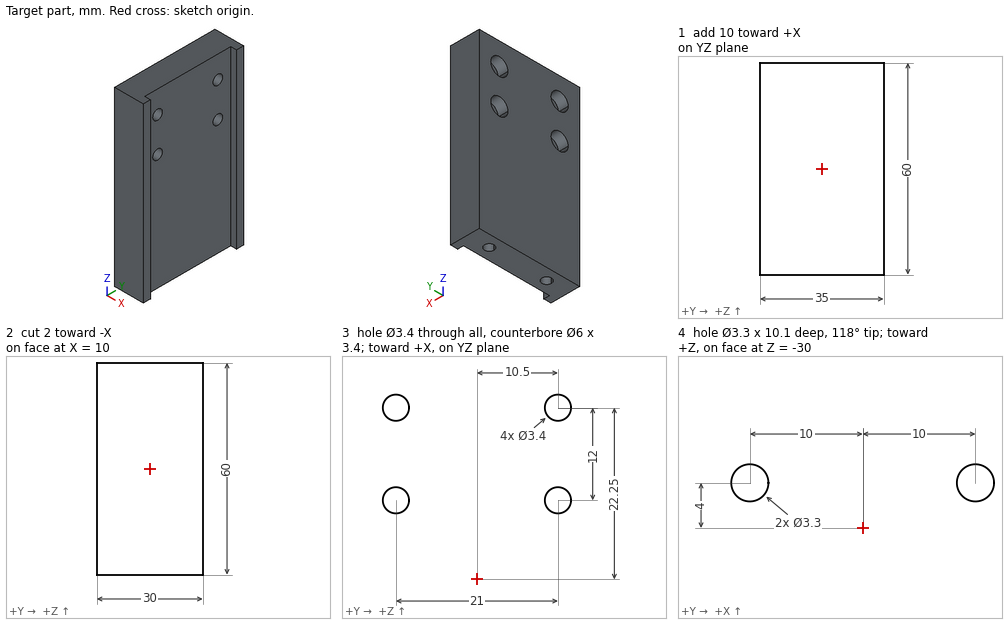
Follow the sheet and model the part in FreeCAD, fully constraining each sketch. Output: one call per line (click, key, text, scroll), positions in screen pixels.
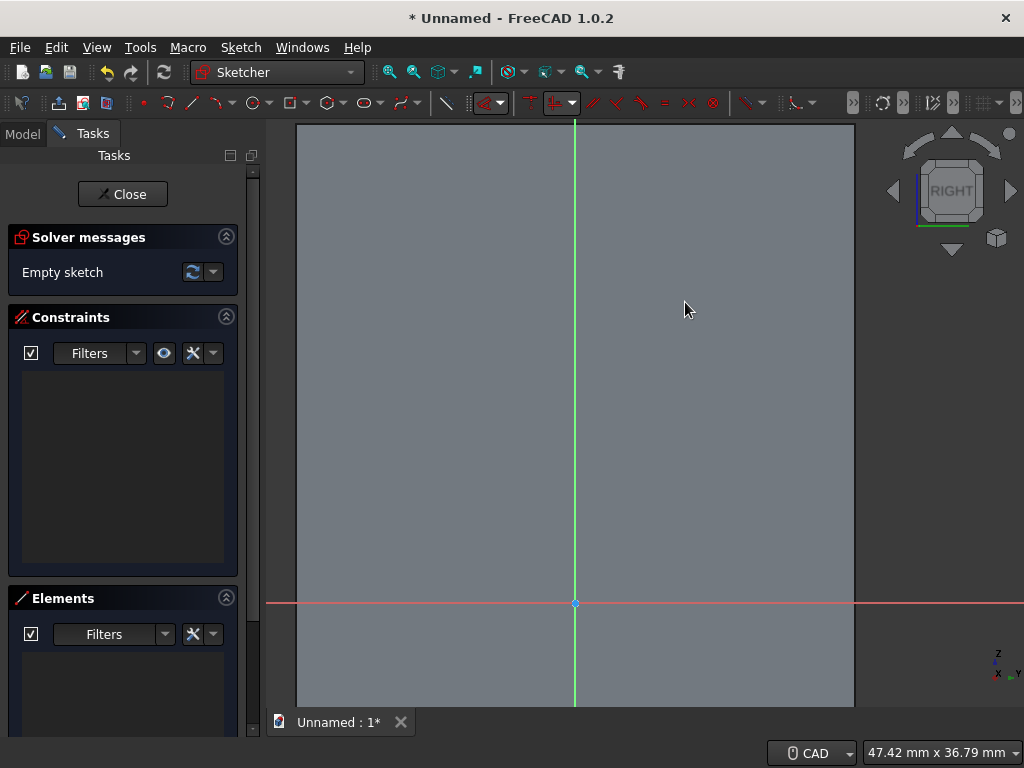
click(254, 104)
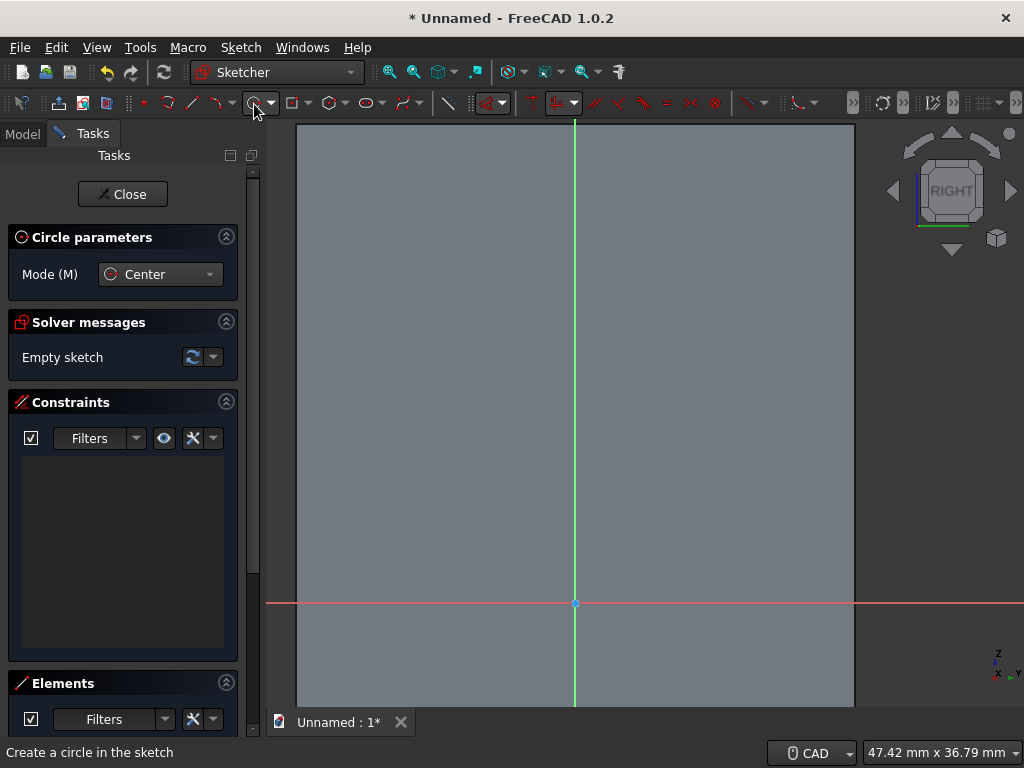
click(743, 248)
move(762, 228)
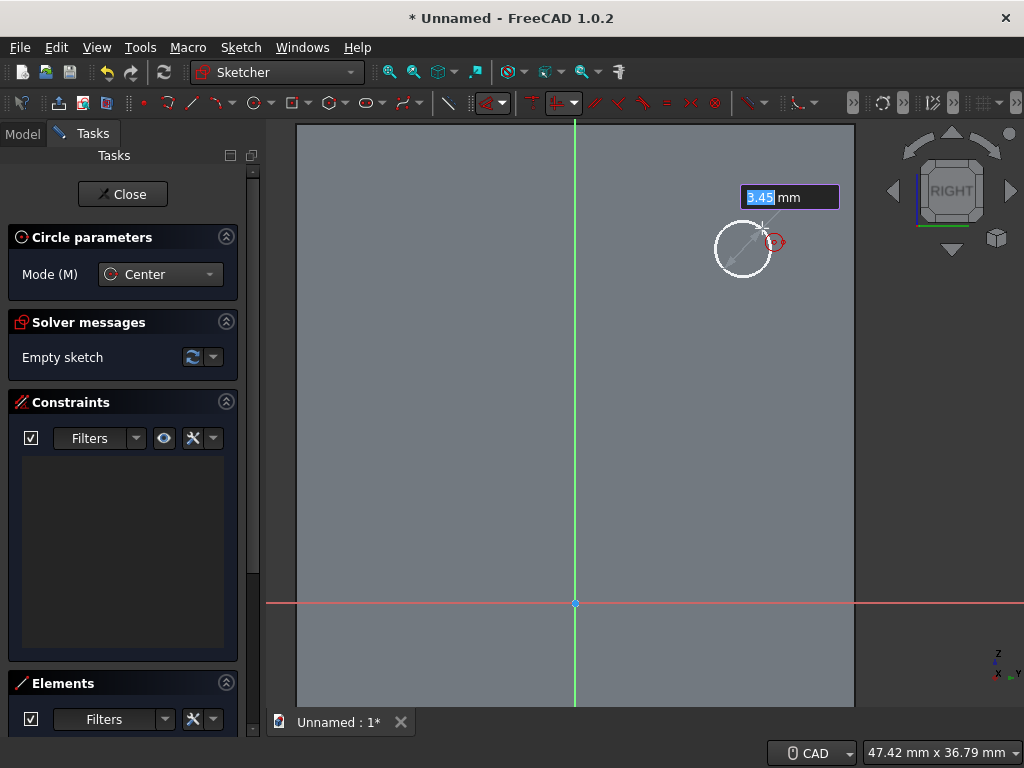
text(3.4)
key(Return)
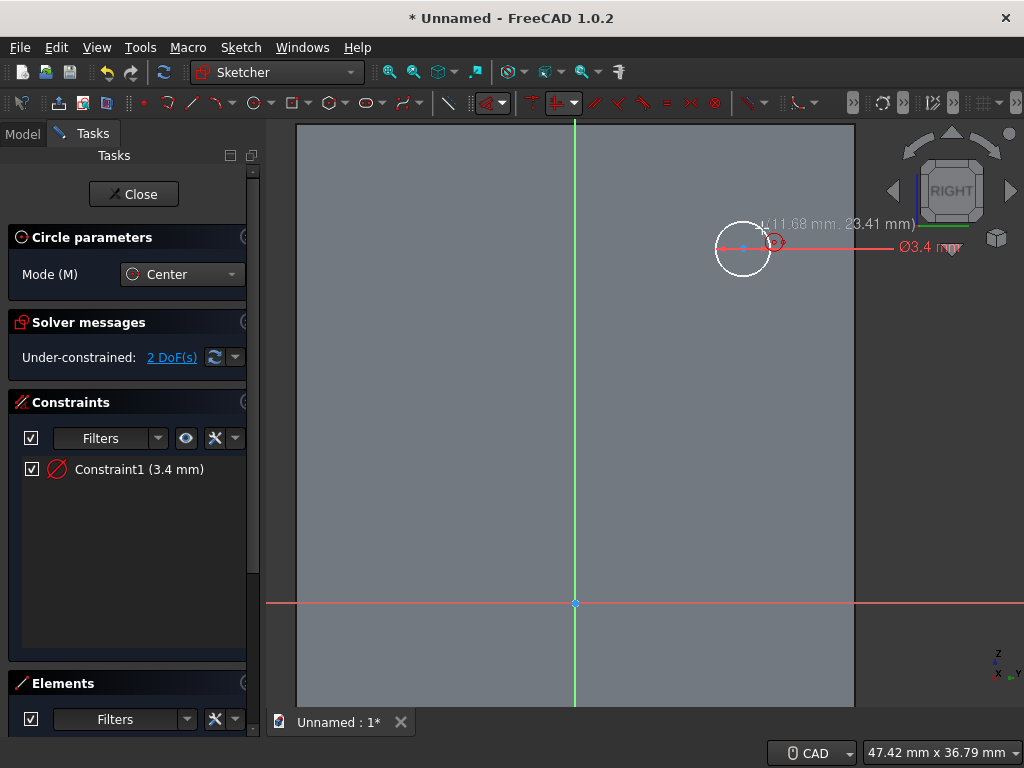
click(743, 439)
move(762, 420)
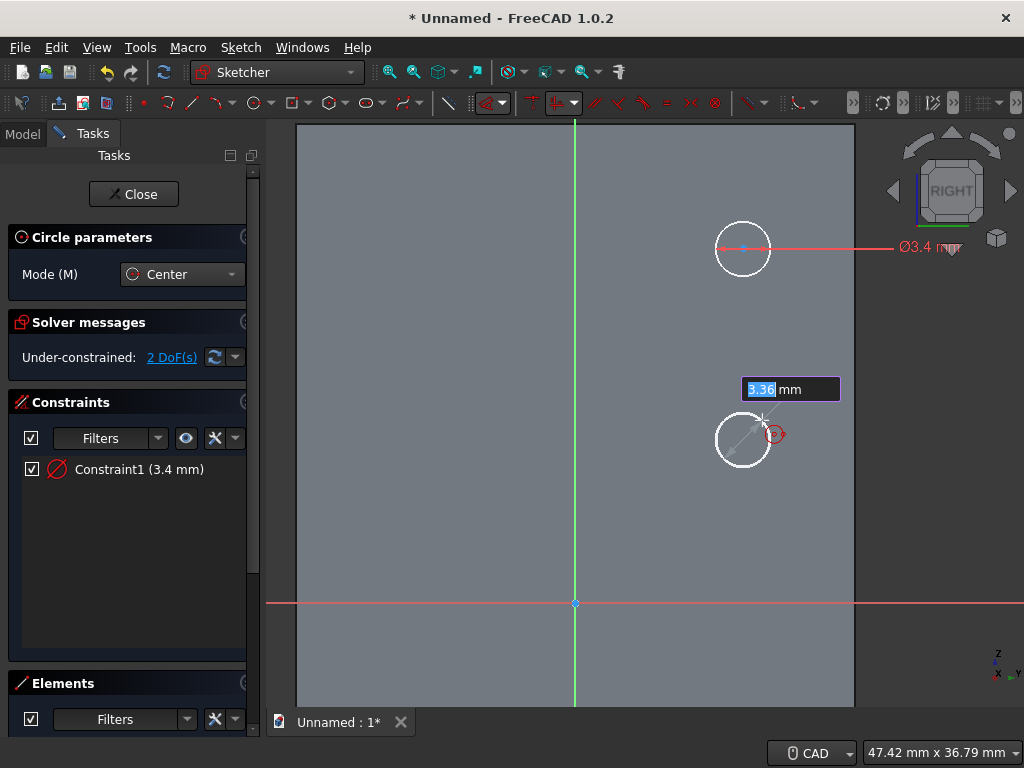
text(3.4)
key(Return)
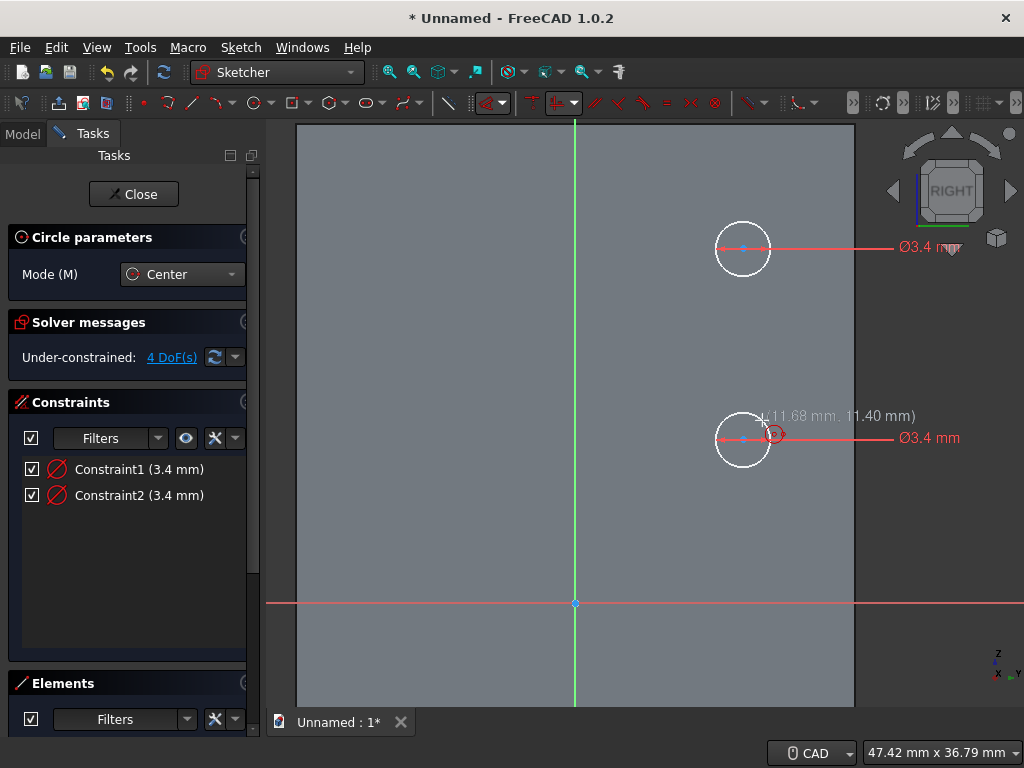
click(407, 439)
move(427, 420)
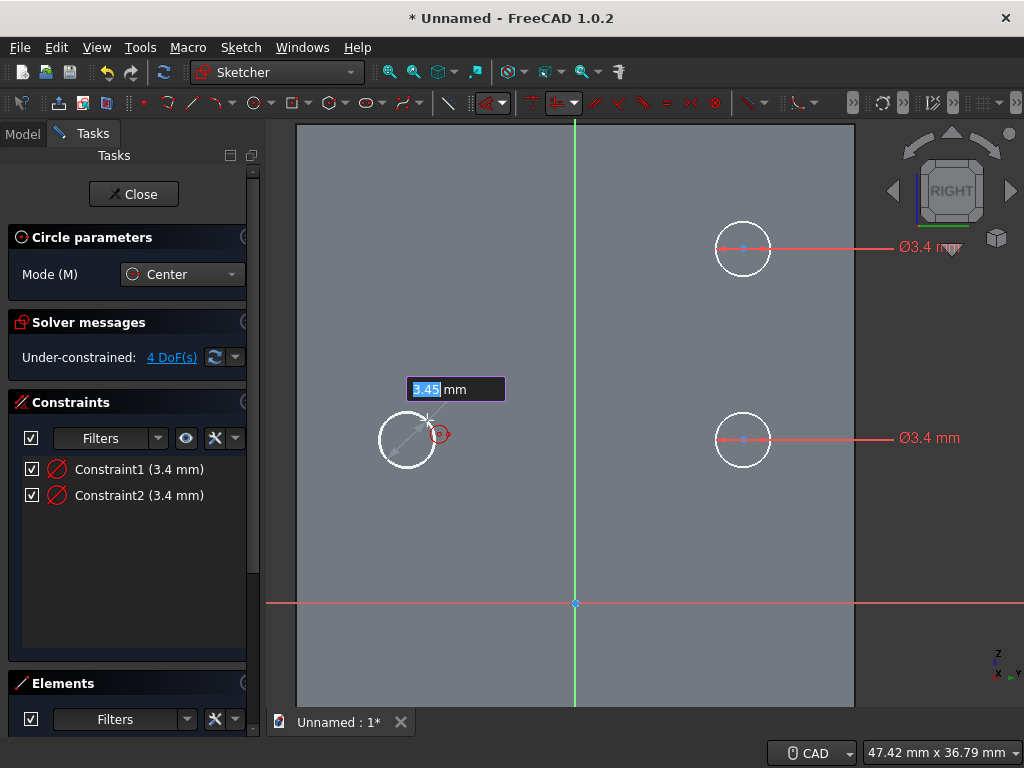
text(3.4)
key(Return)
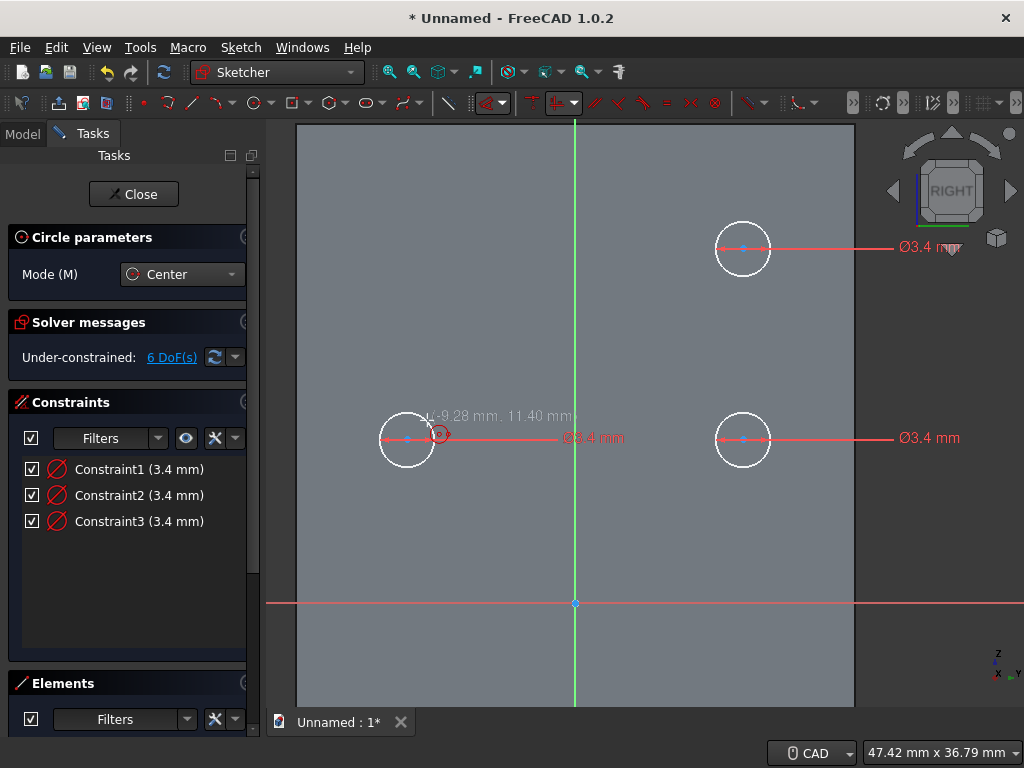
click(407, 248)
move(427, 228)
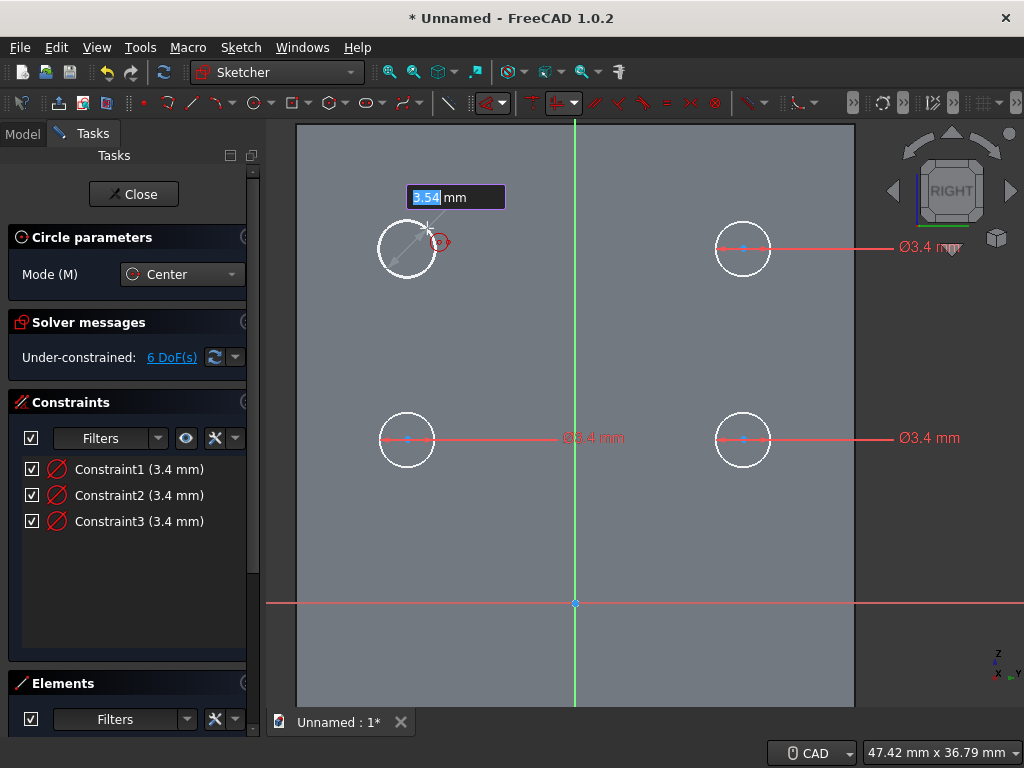
text(3.4)
key(Return)
key(Escape)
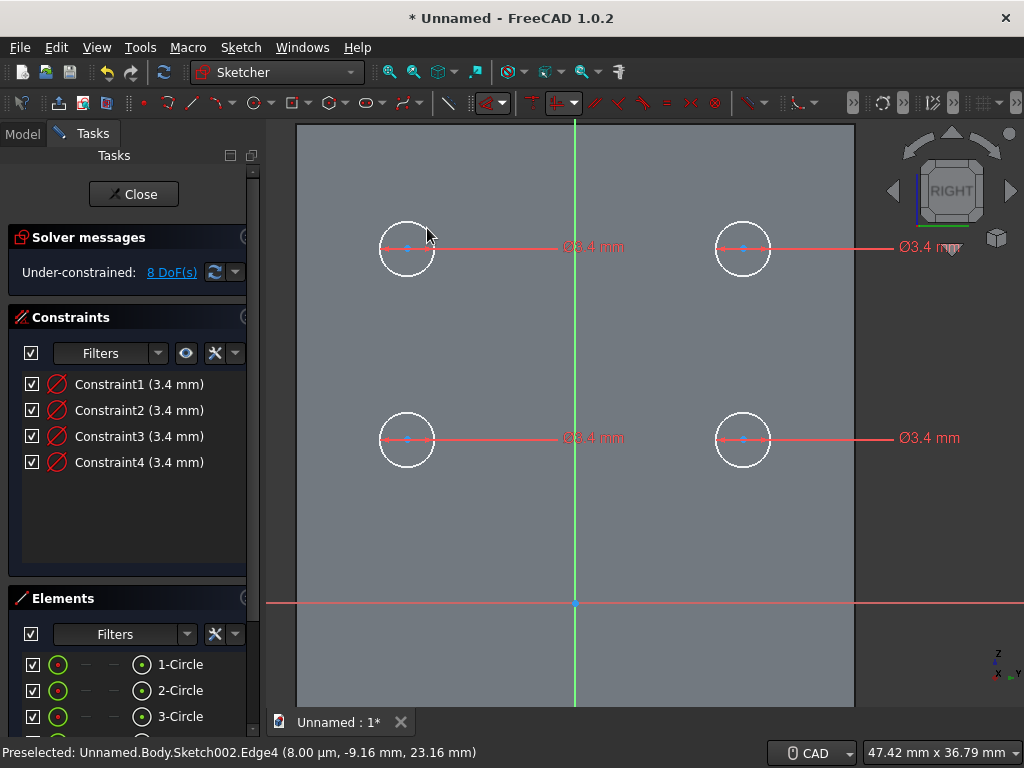
click(743, 249)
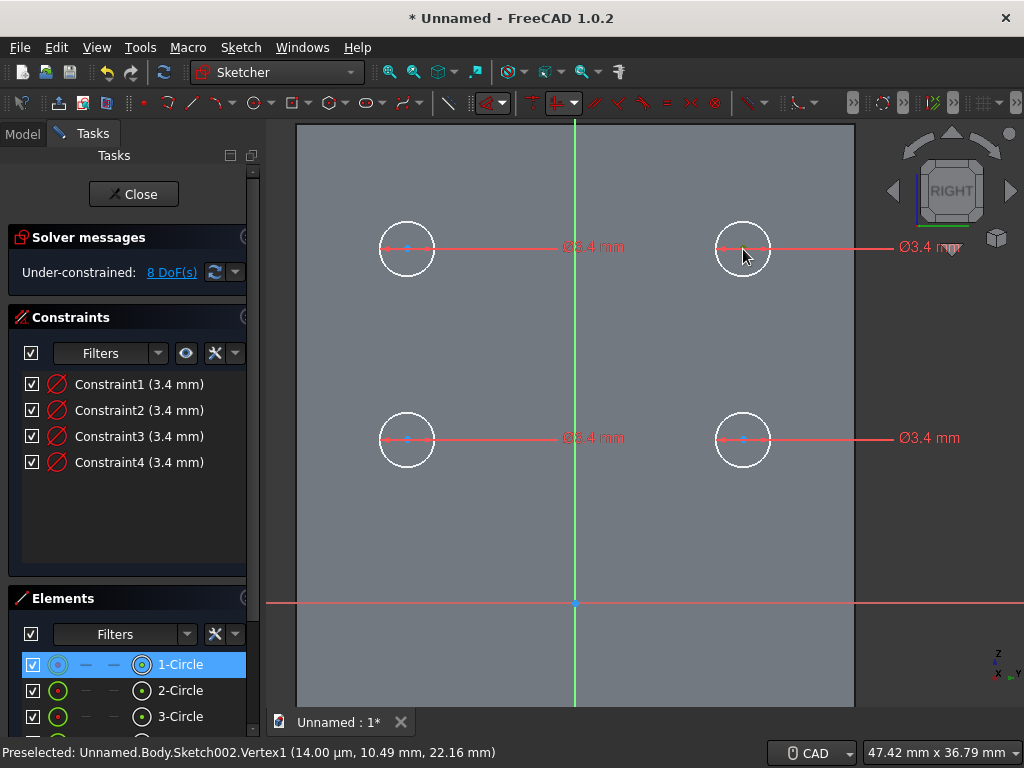
click(743, 440)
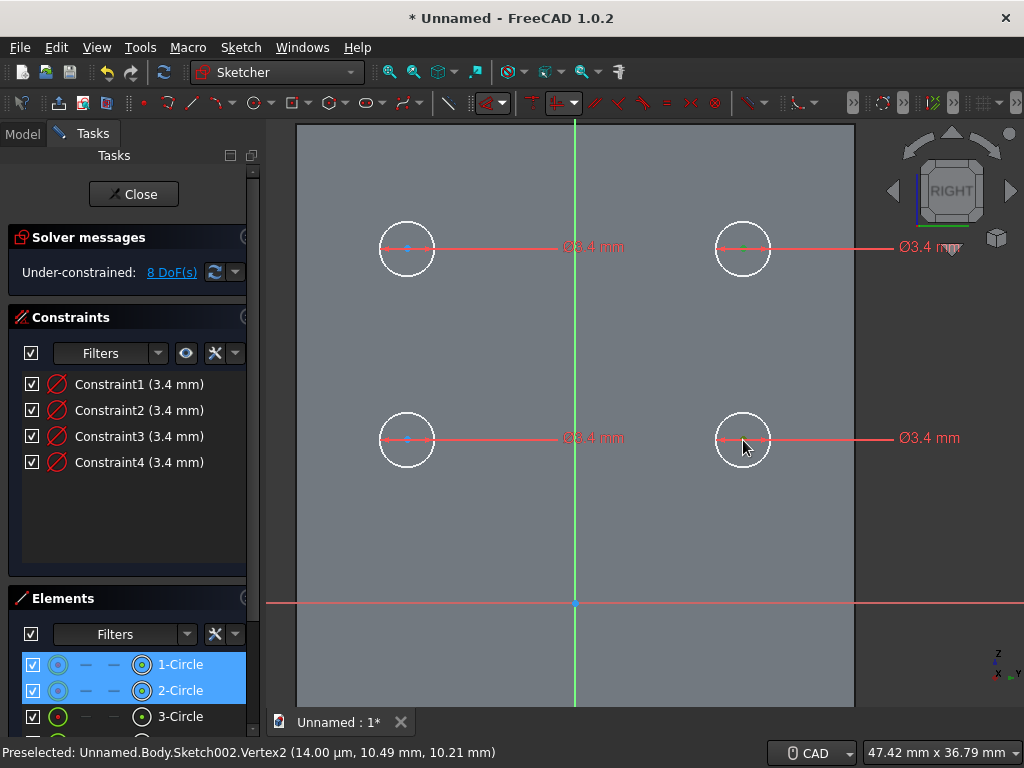
key(v)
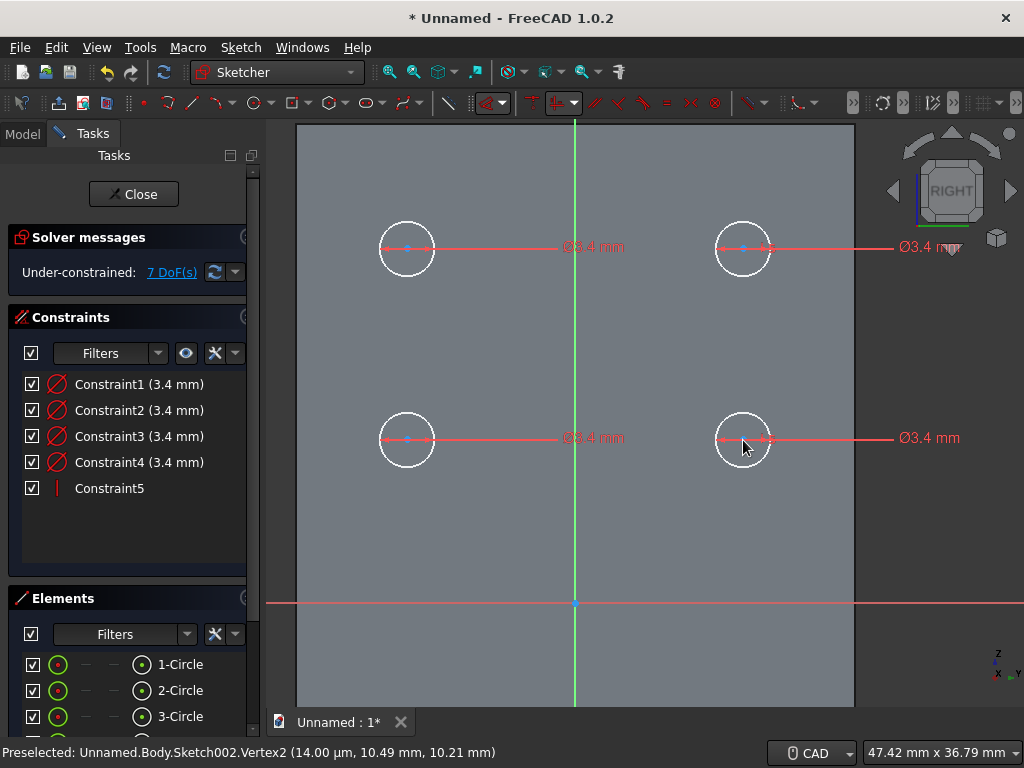
click(743, 440)